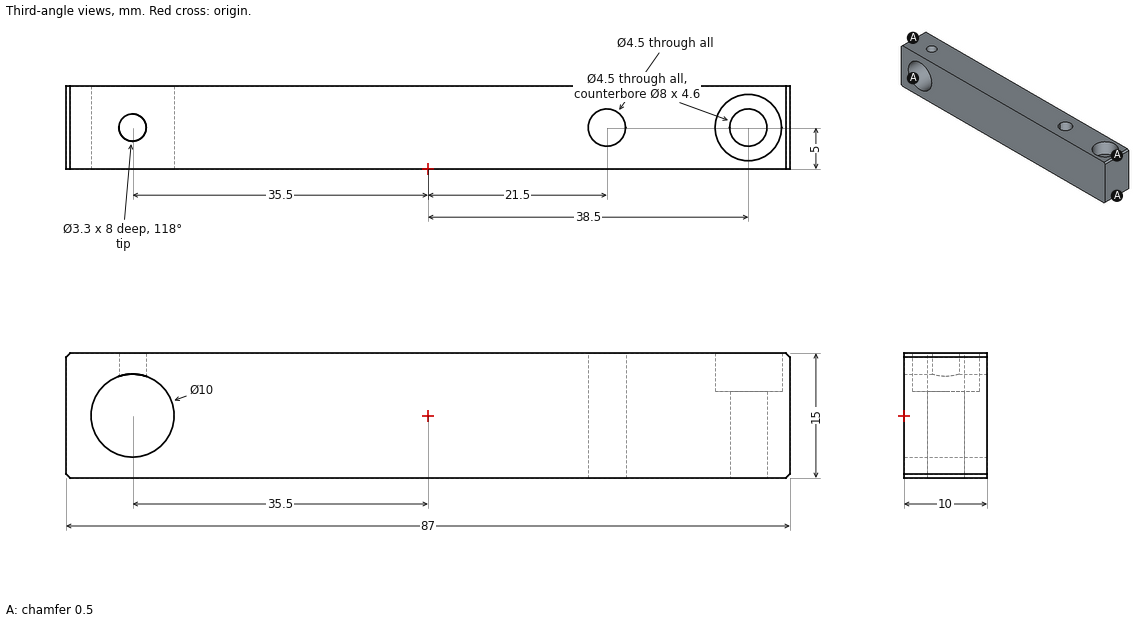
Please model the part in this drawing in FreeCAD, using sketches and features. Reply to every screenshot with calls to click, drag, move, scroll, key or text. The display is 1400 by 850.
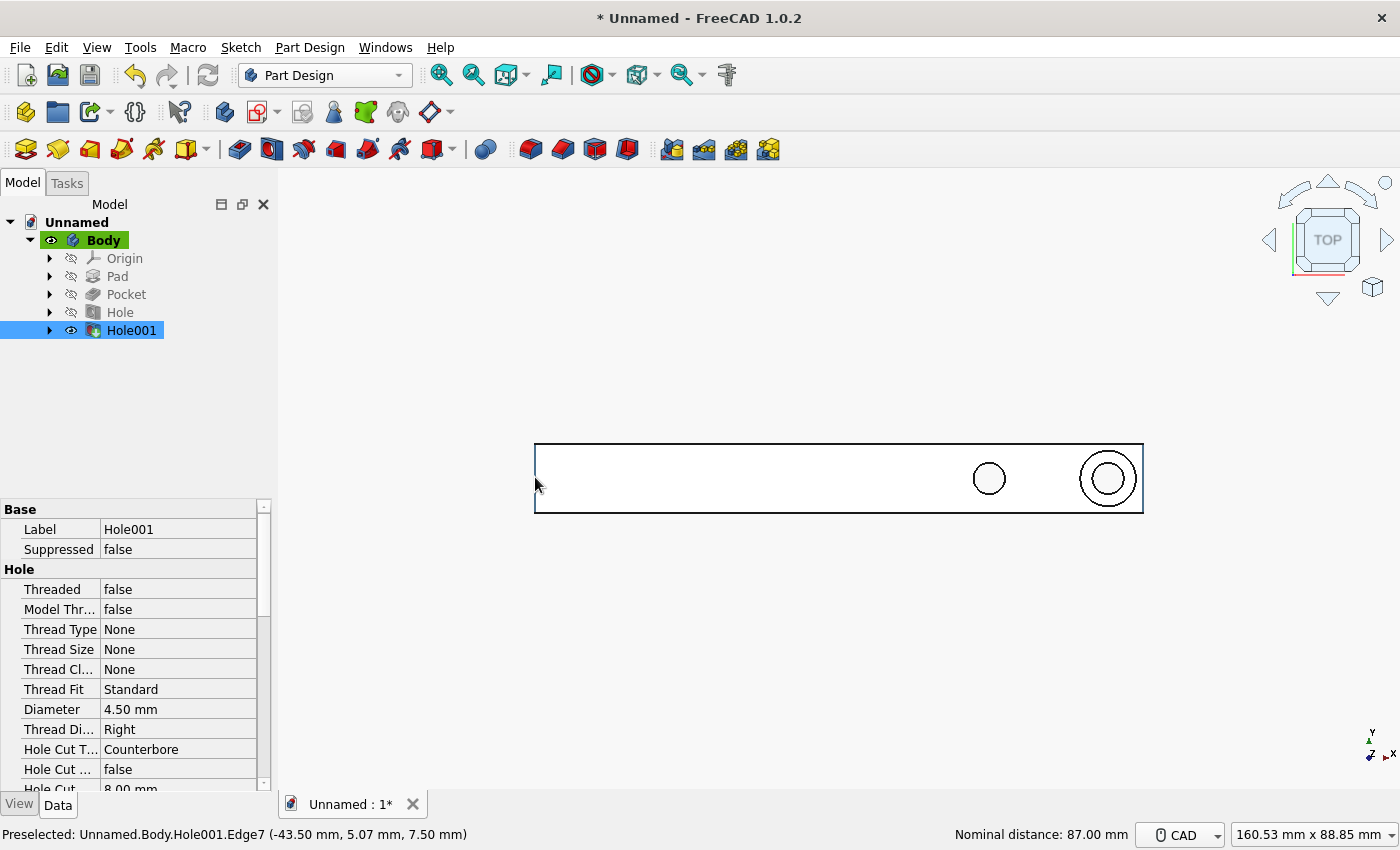
key(0)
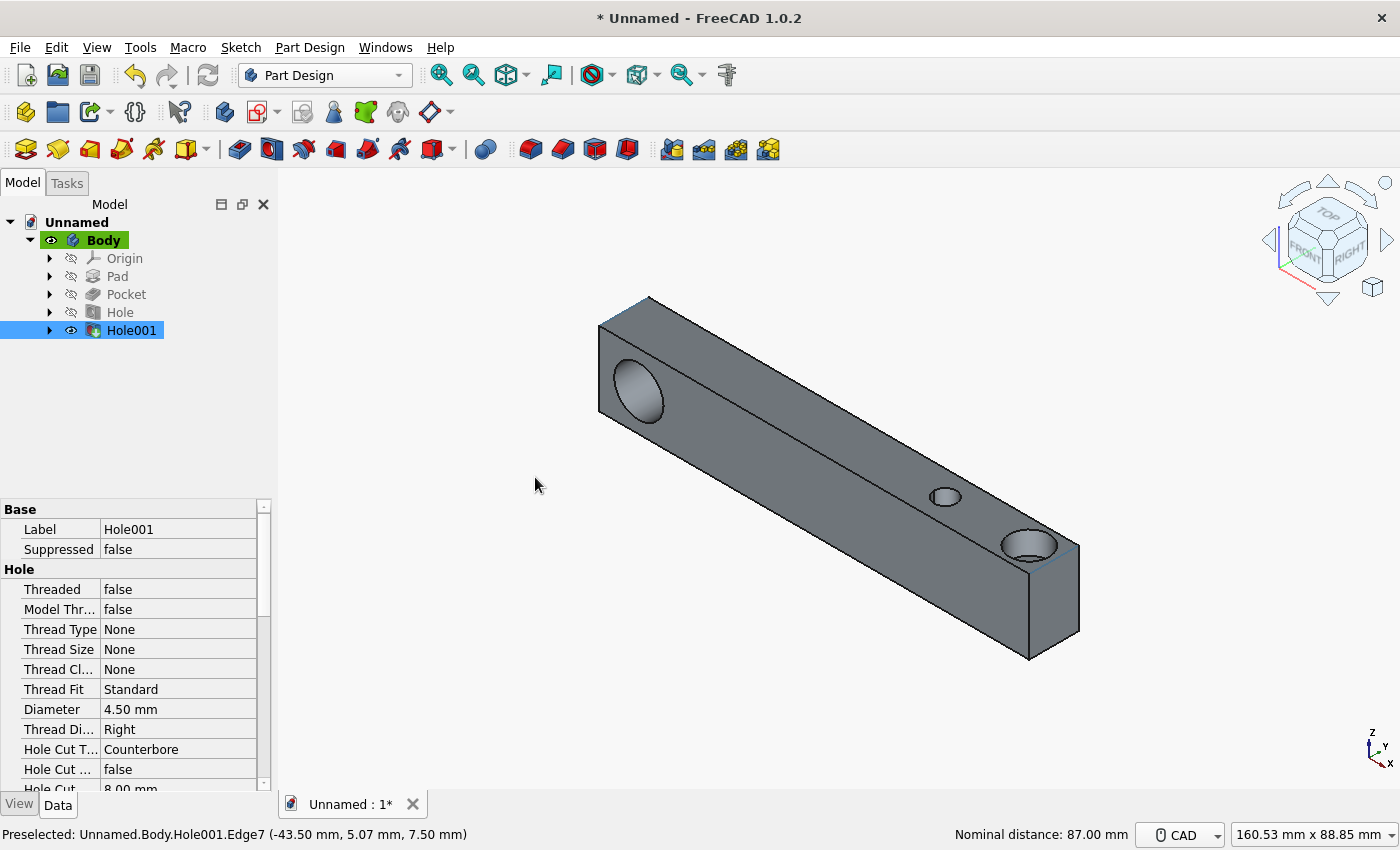
key(1)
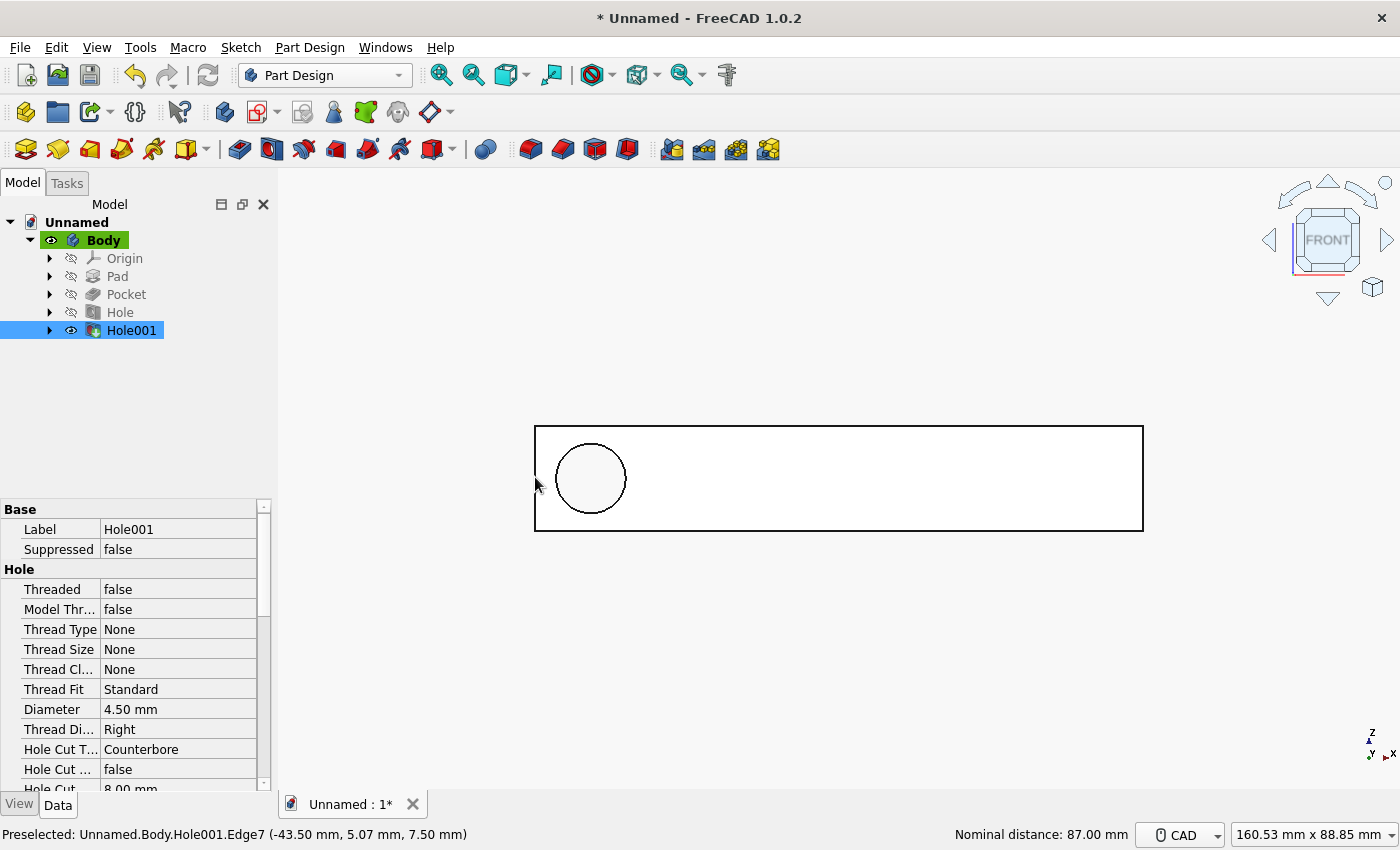
key(3)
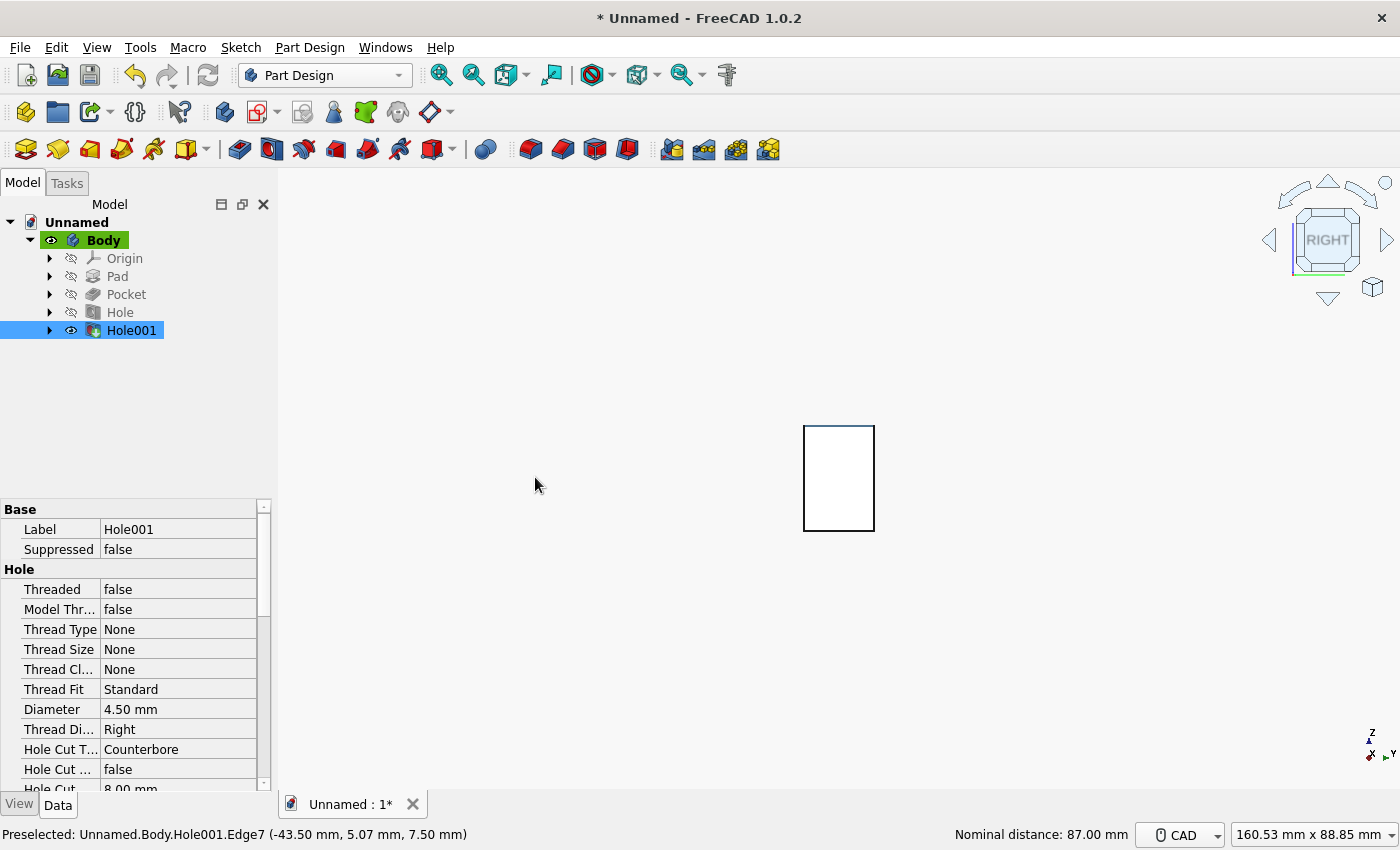
click(442, 76)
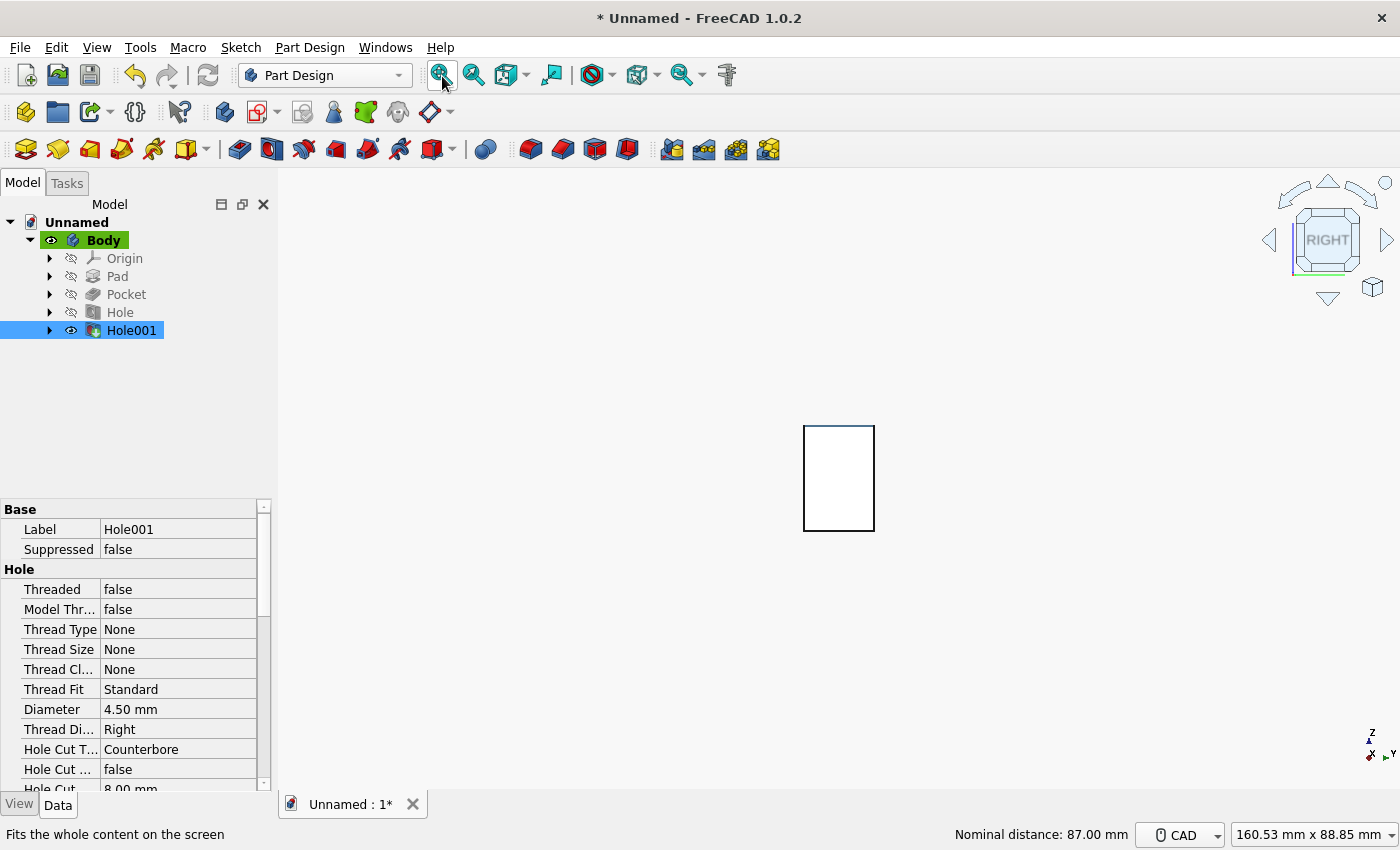
click(839, 530, ctrl)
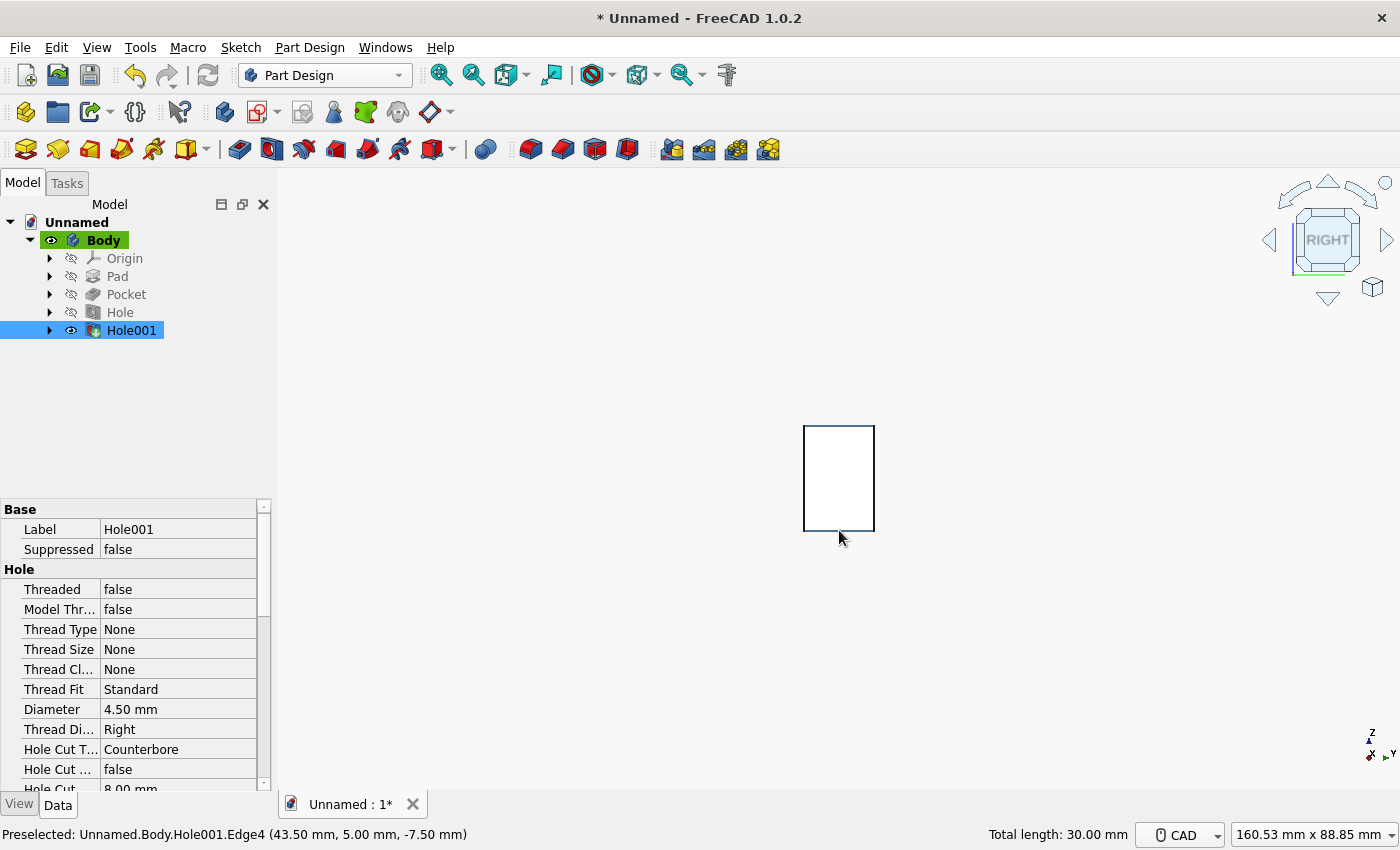
key(5)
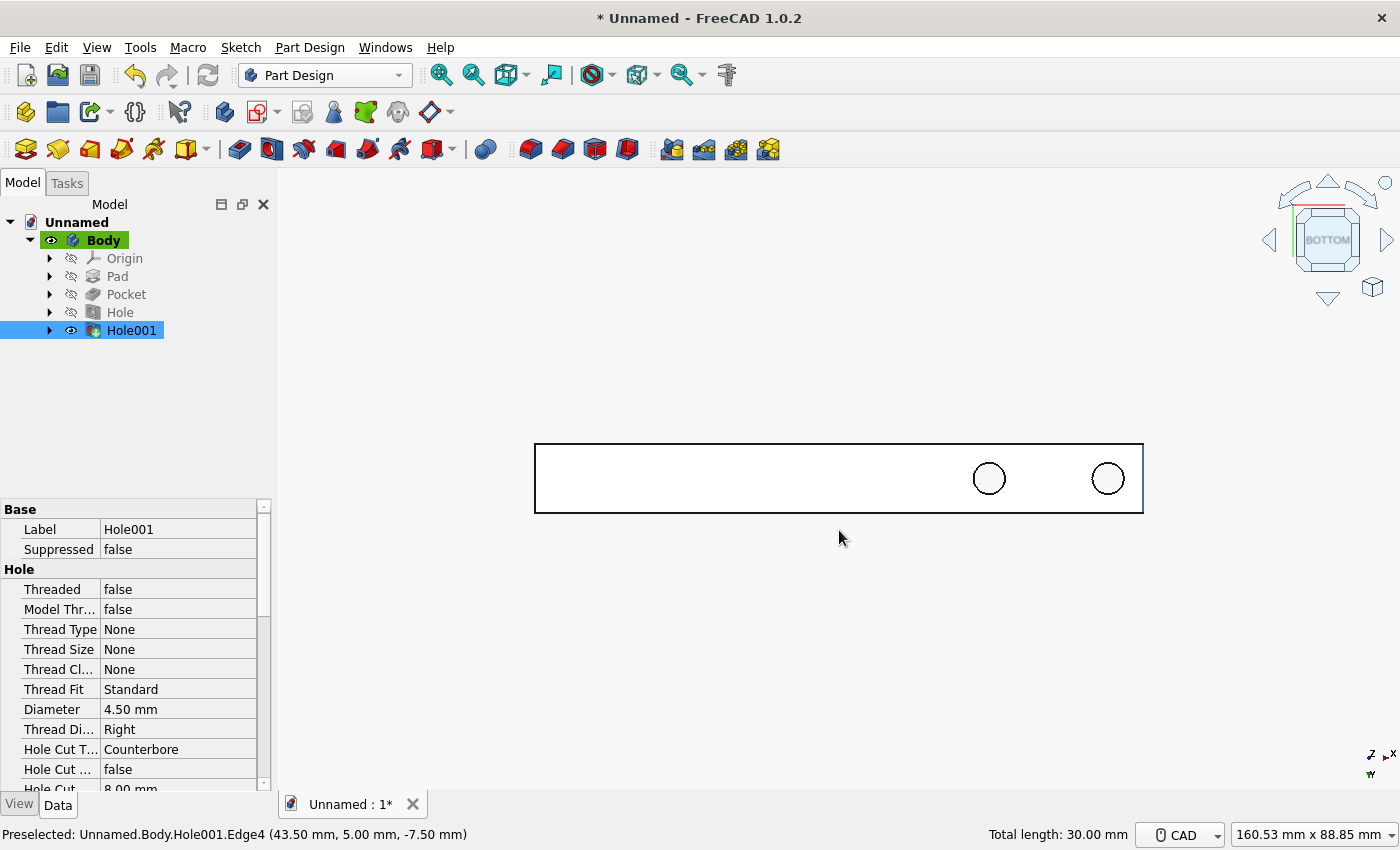
click(535, 477, ctrl)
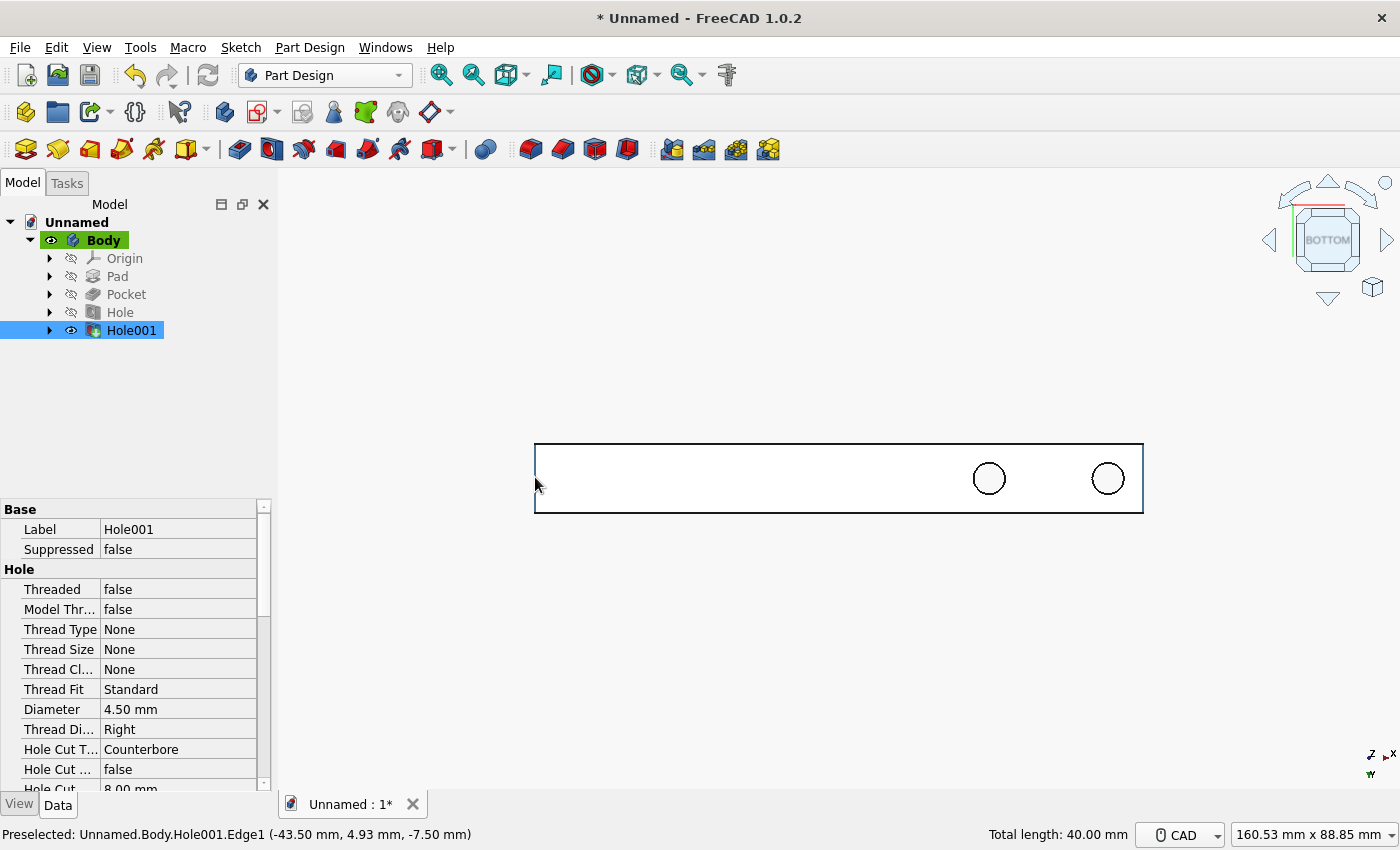
click(564, 150)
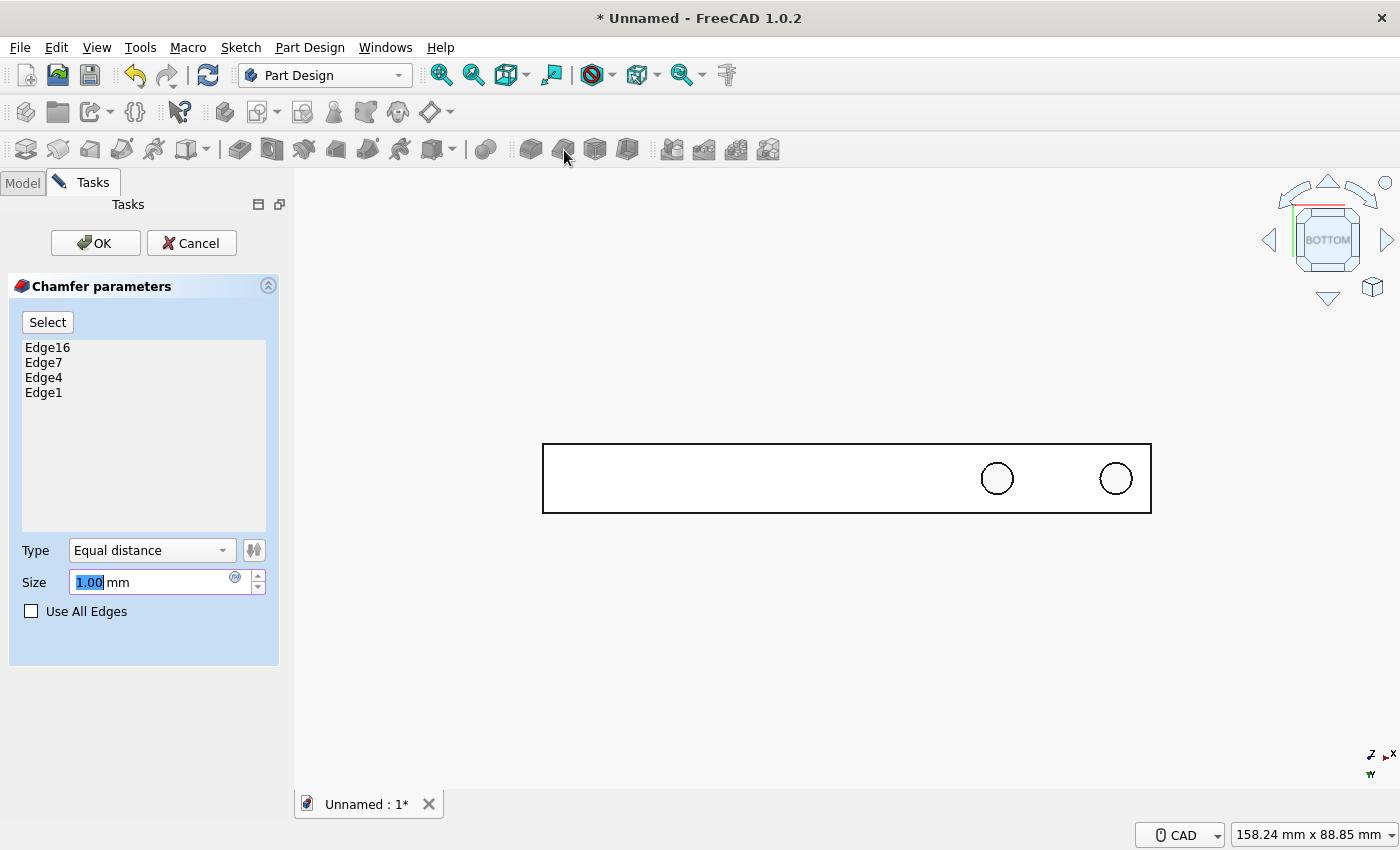
text(0.5)
key(Tab)